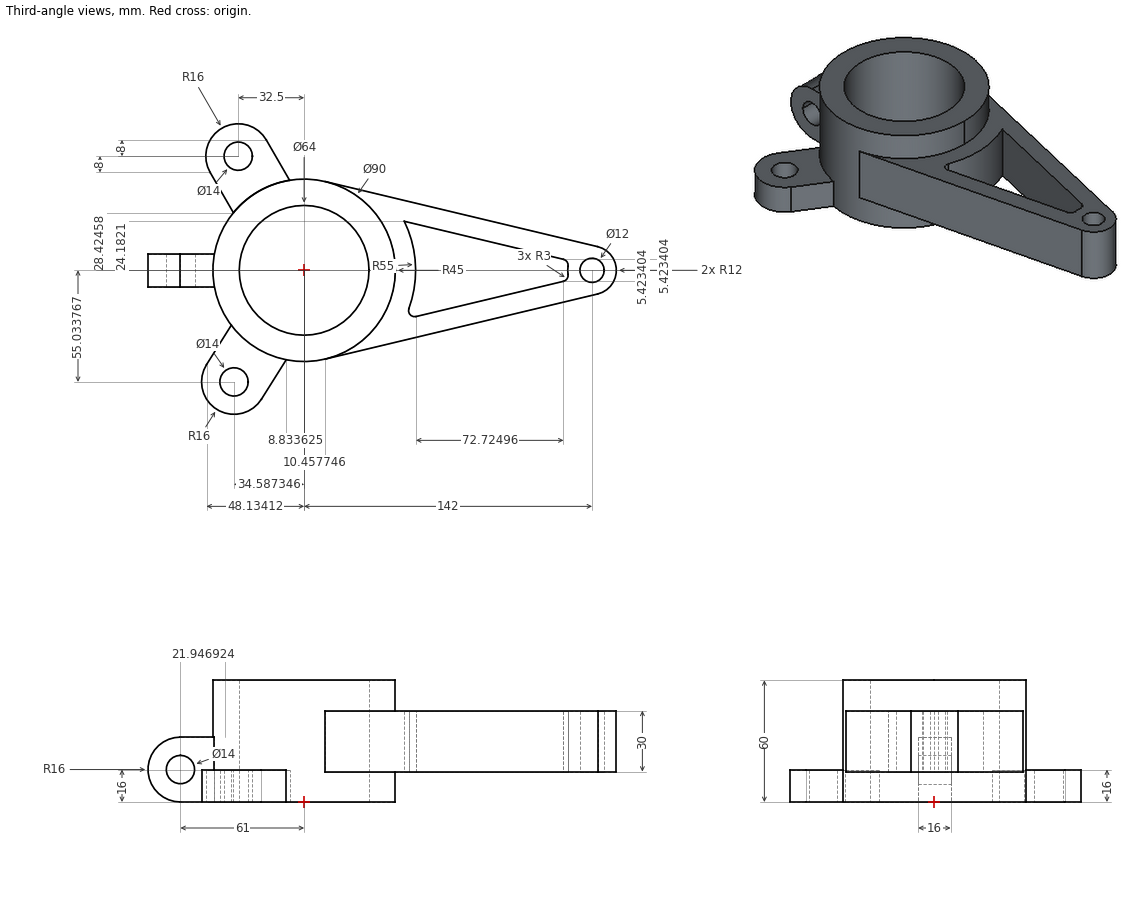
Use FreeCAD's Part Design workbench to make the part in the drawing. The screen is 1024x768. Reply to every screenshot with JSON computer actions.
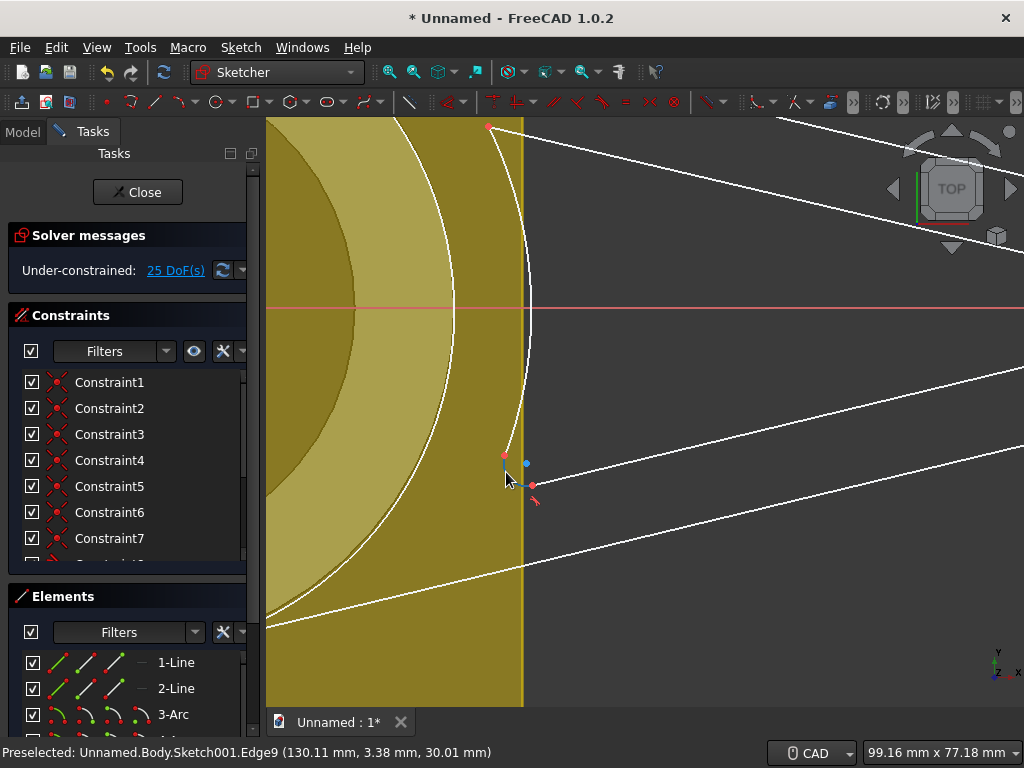
{"action": "left_click", "coordinate": [505, 470]}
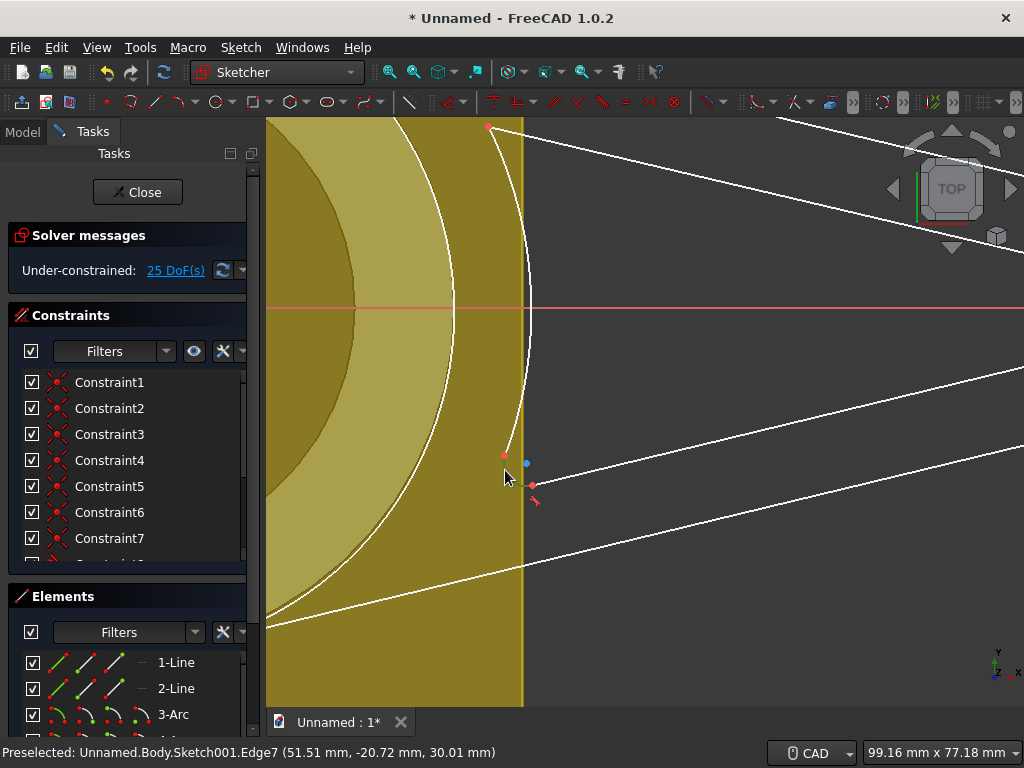
{"action": "left_click", "coordinate": [529, 357]}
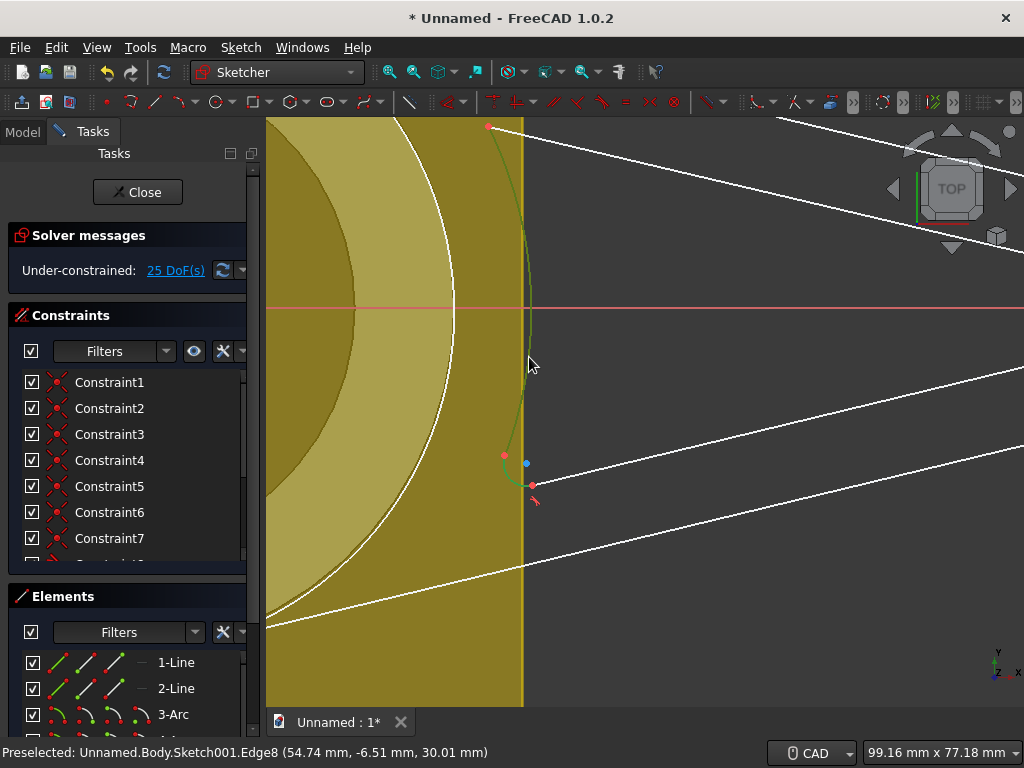
{"action": "key", "text": "t"}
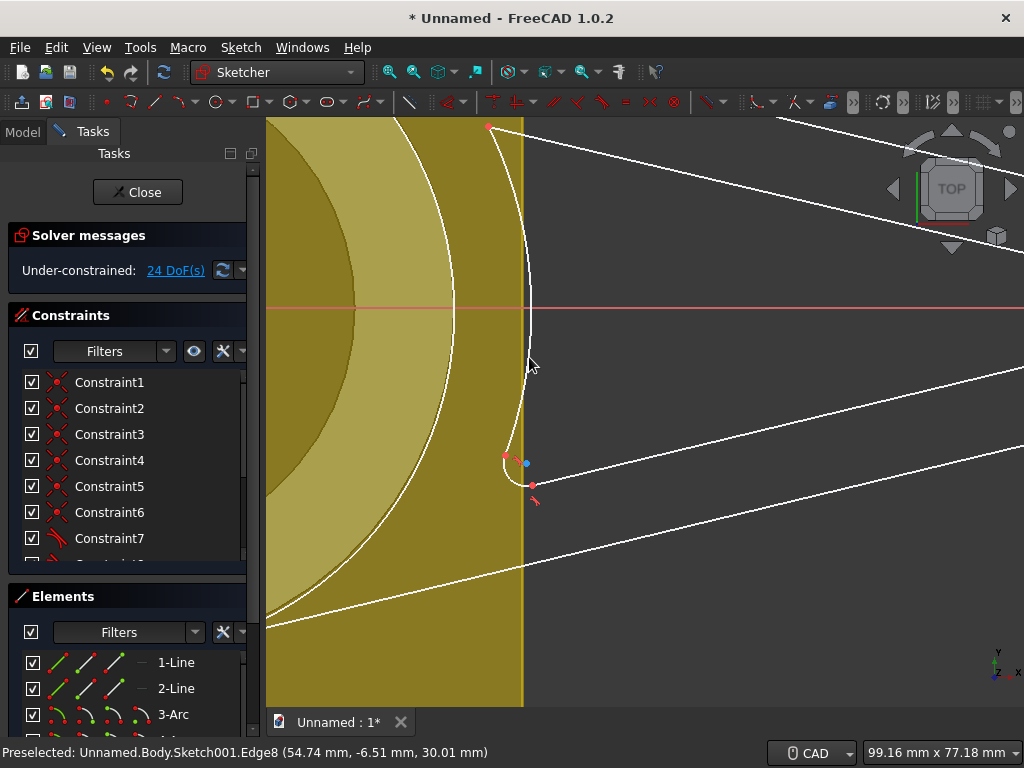
{"action": "scroll", "coordinate": [505, 472], "scroll_direction": "down", "scroll_amount": 5}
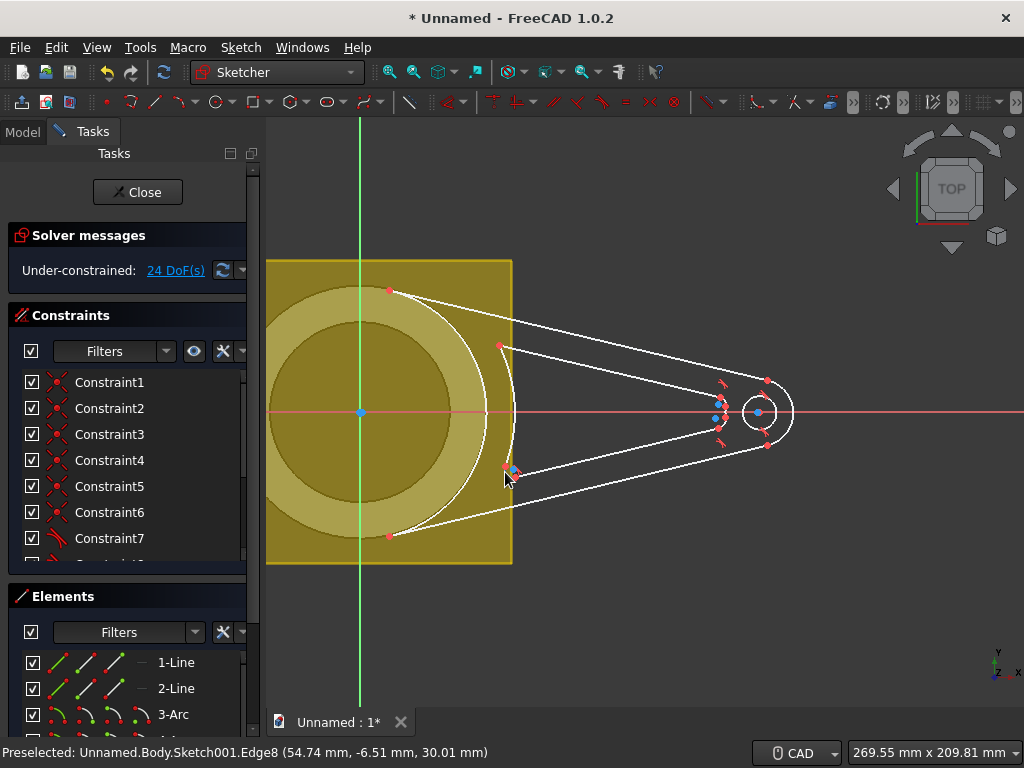
{"action": "scroll", "coordinate": [726, 403], "scroll_direction": "up", "scroll_amount": 7}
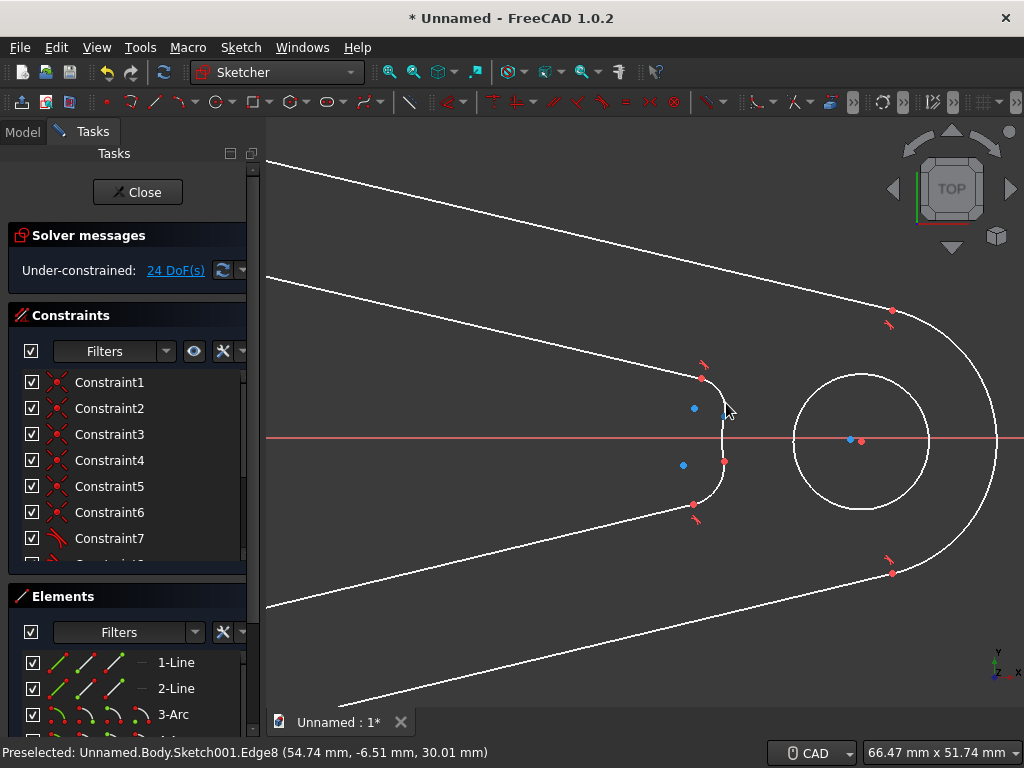
{"action": "left_click", "coordinate": [724, 402]}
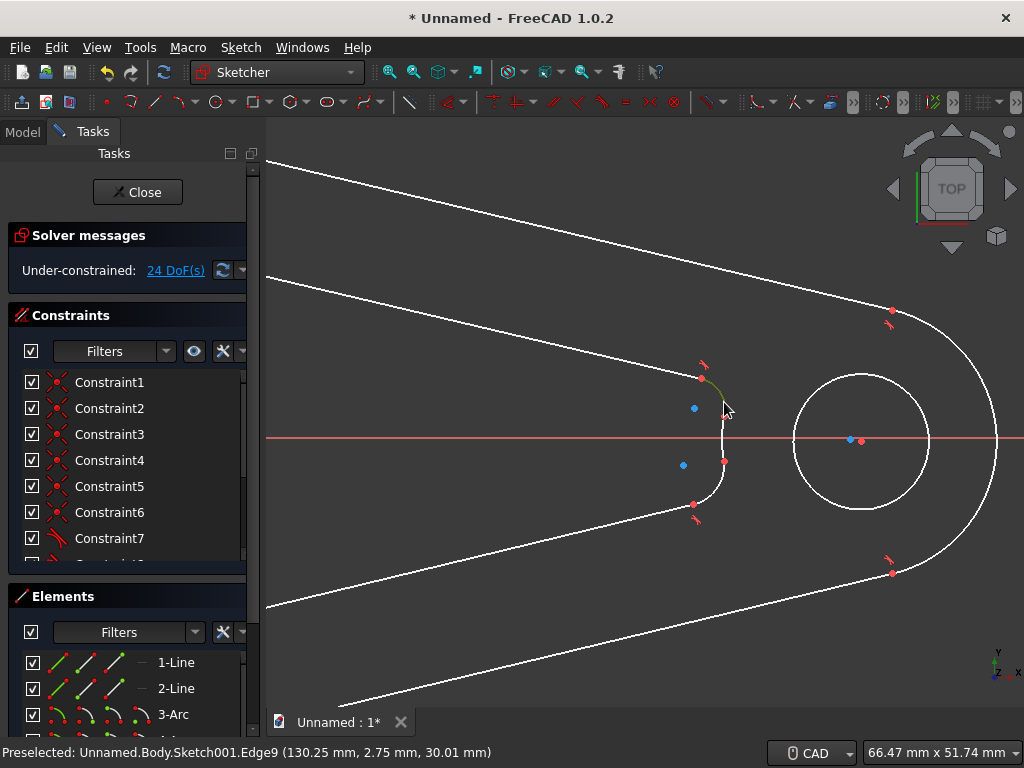
{"action": "scroll", "coordinate": [722, 448], "scroll_direction": "up", "scroll_amount": 2}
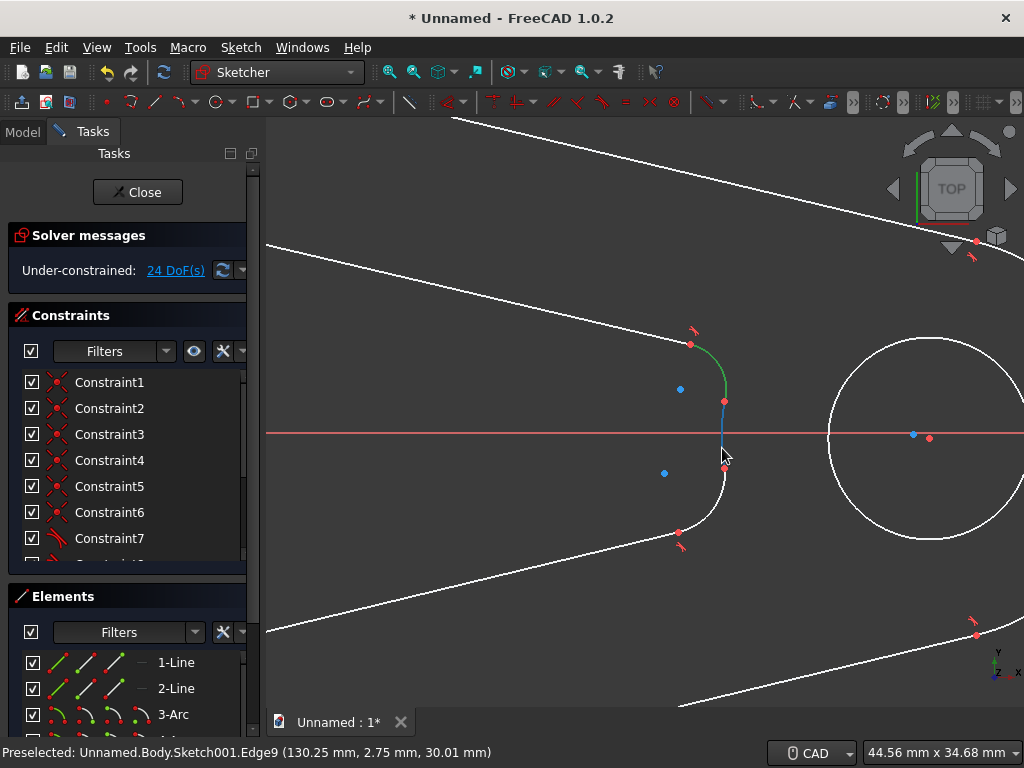
{"action": "left_click", "coordinate": [722, 448]}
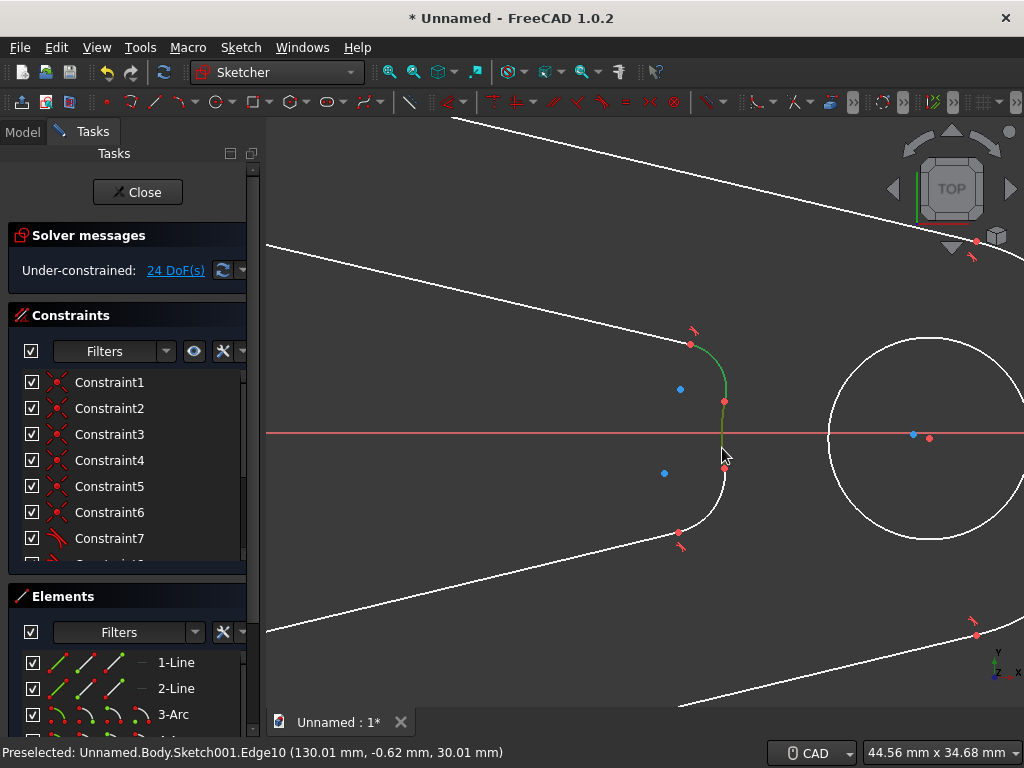
{"action": "key", "text": "t"}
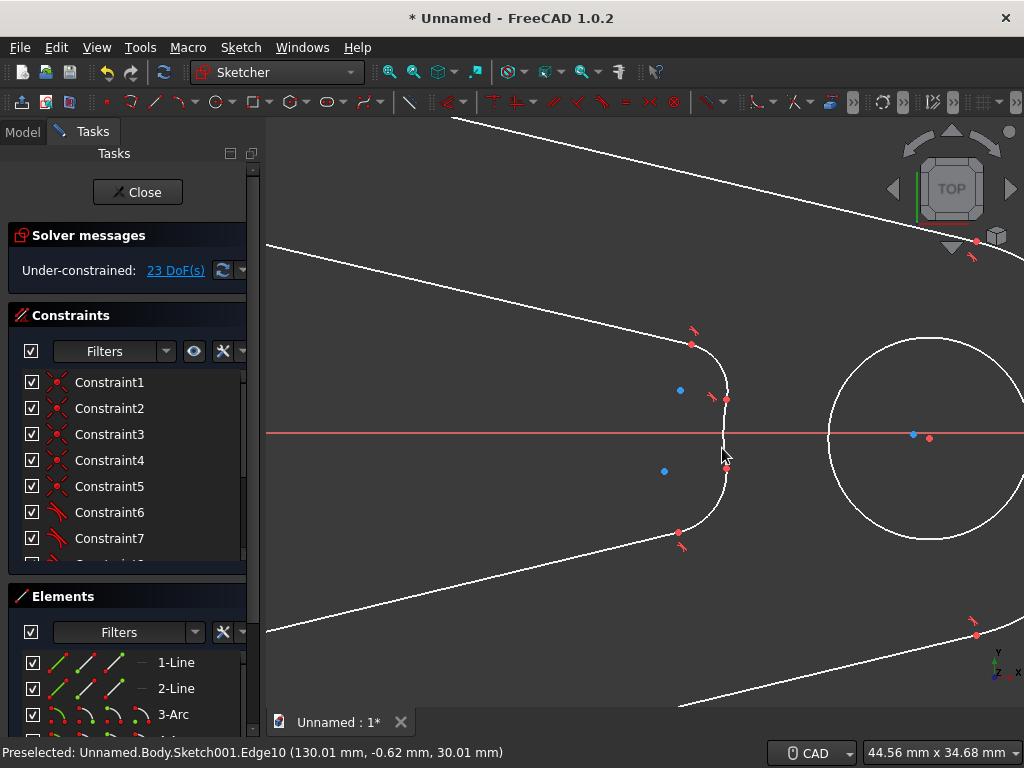
{"action": "left_click", "coordinate": [724, 420]}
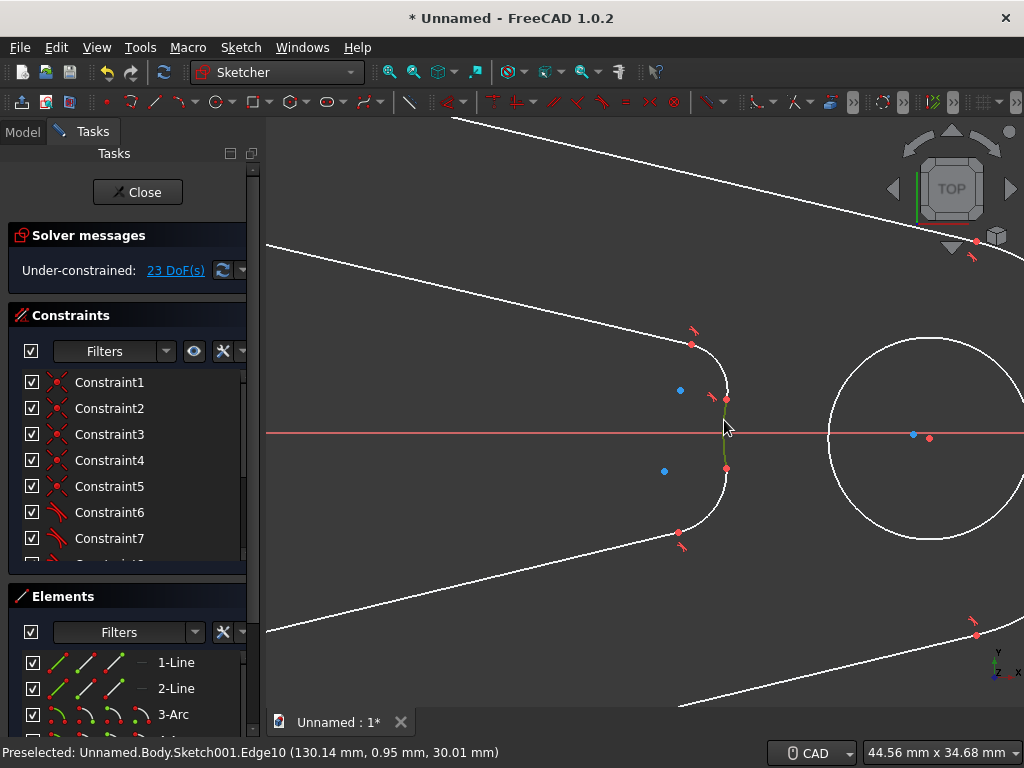
{"action": "left_click", "coordinate": [702, 521]}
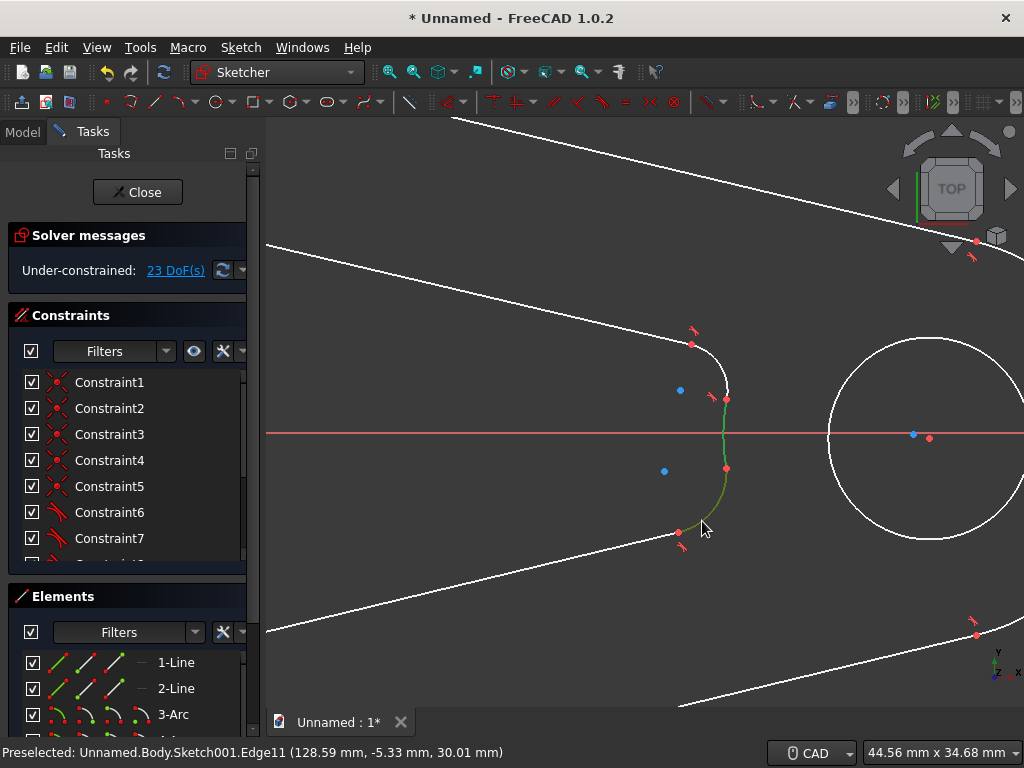
{"action": "left_click", "coordinate": [602, 102]}